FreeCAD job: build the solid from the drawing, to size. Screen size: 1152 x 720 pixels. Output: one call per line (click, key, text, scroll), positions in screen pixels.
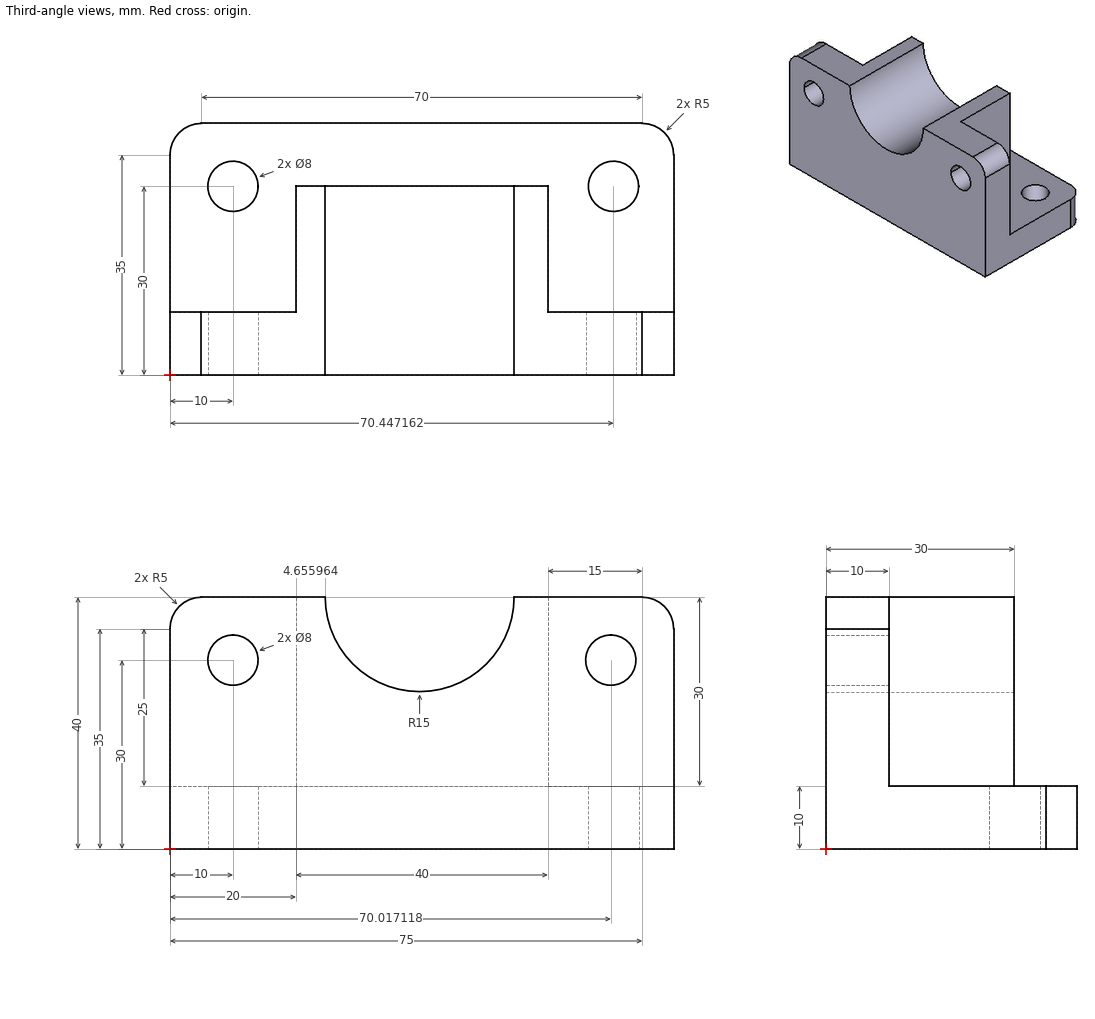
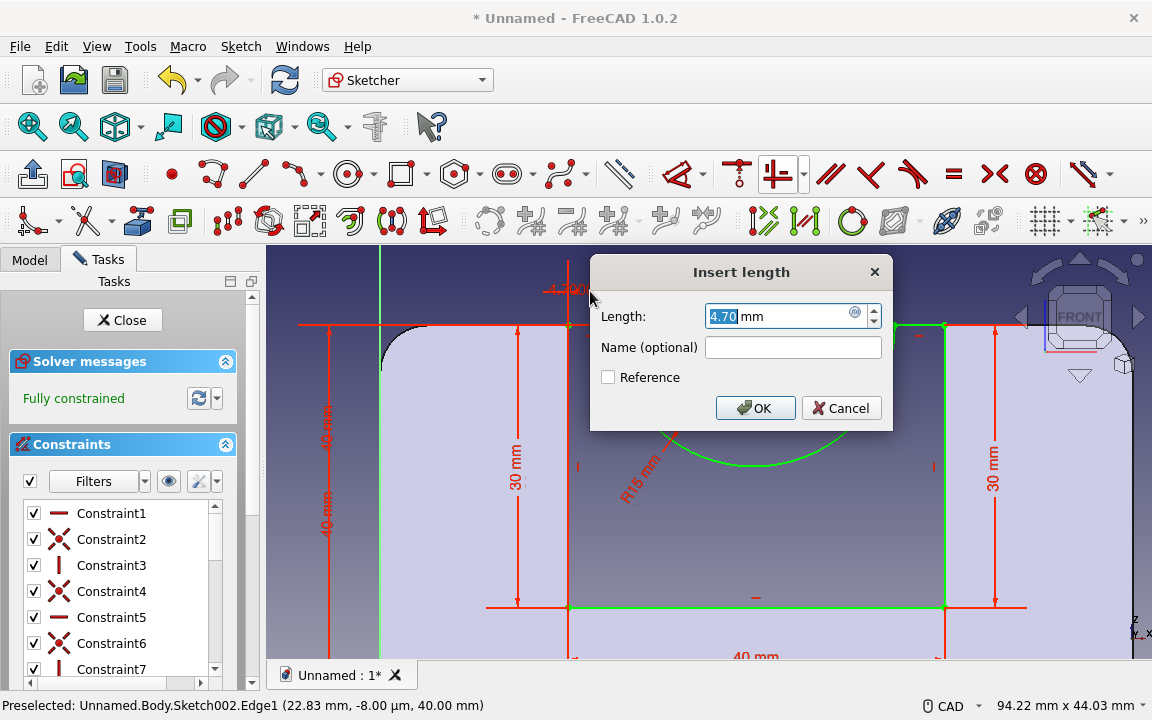
text(4.655964)
key(Return)
key(Escape)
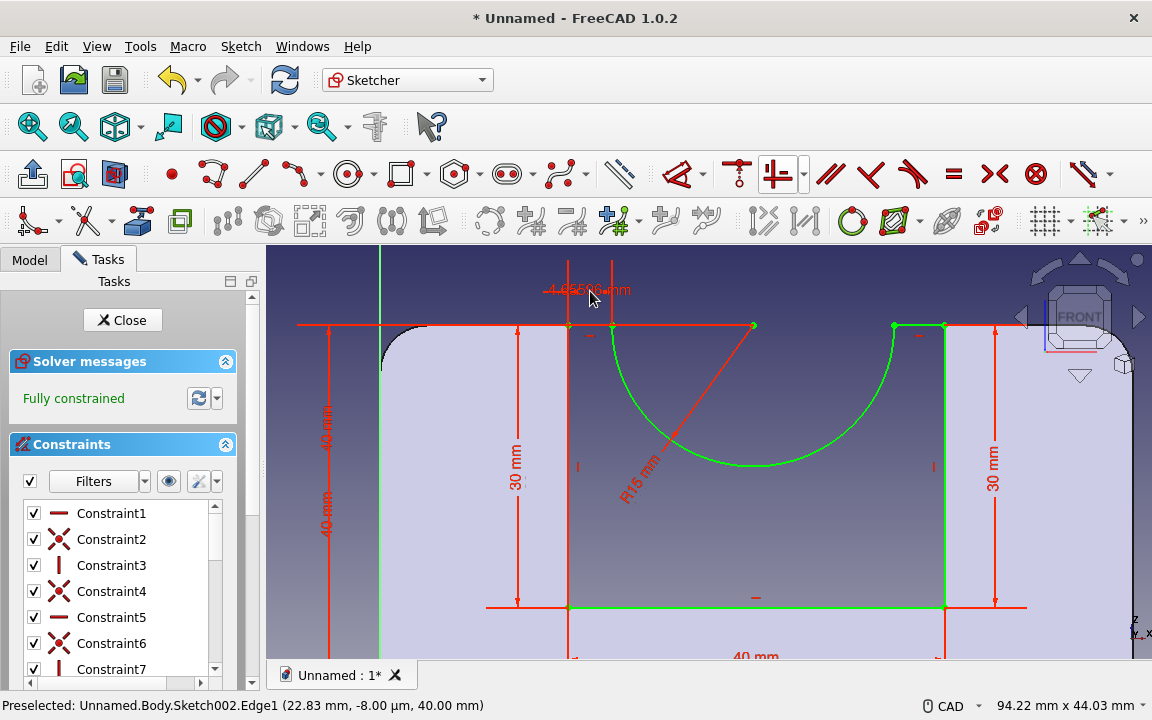
click(123, 320)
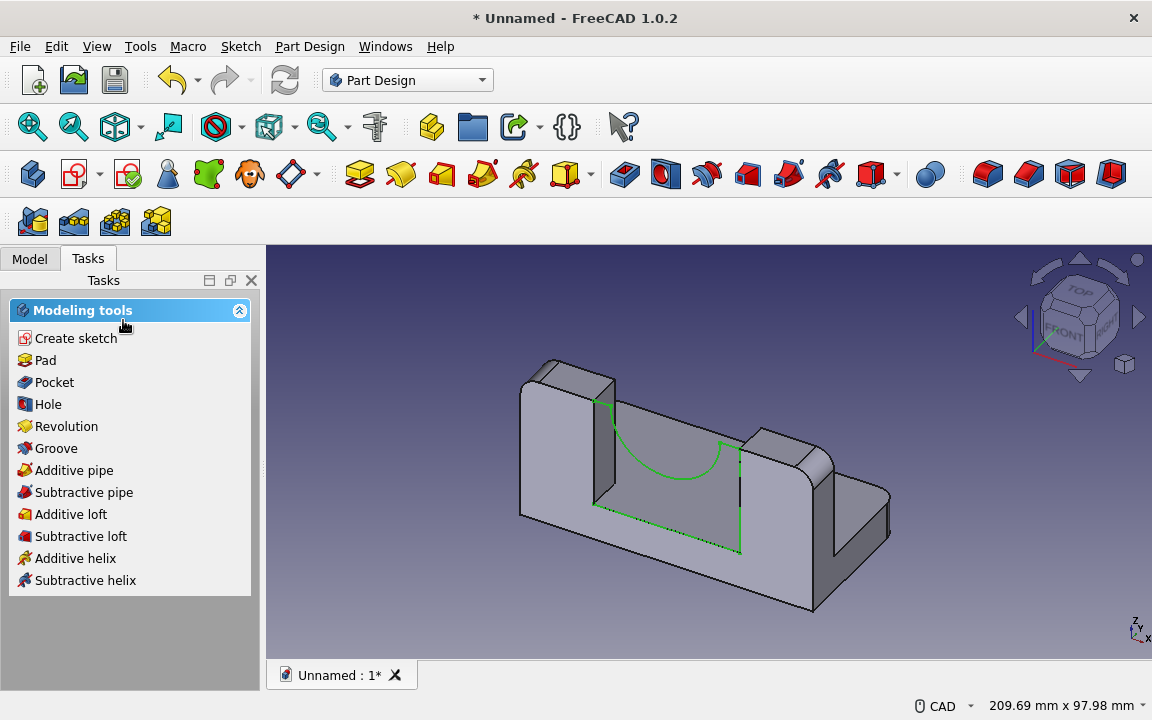
click(360, 174)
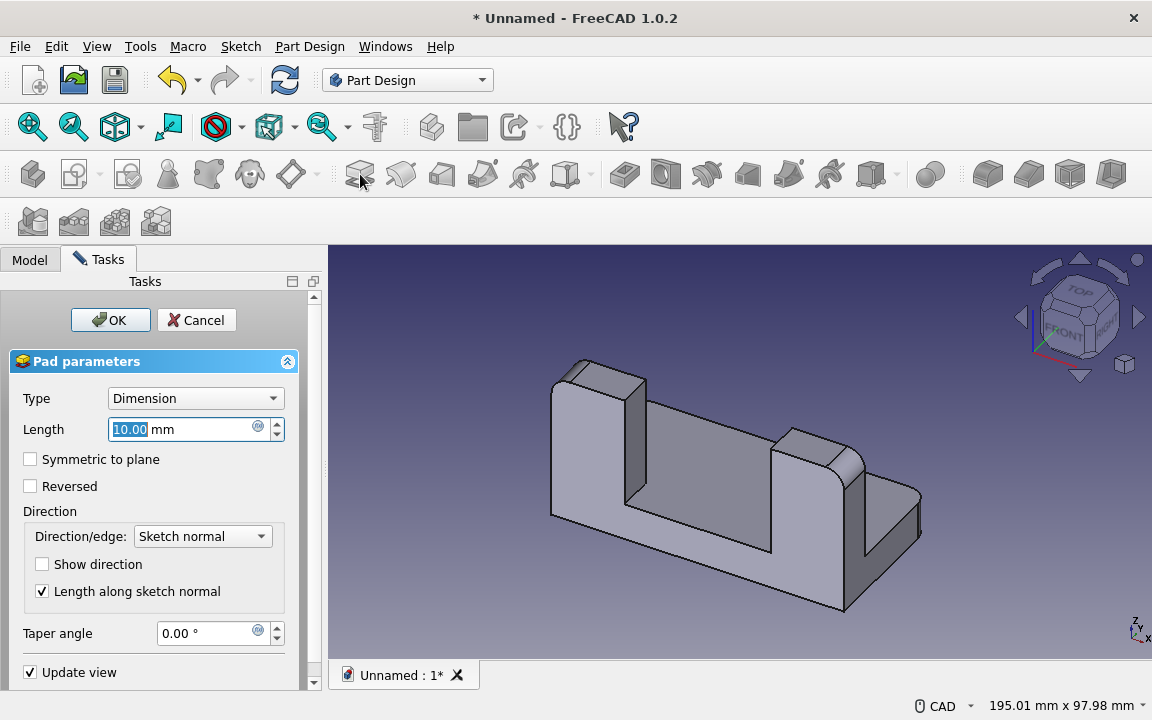
text(30)
key(Tab)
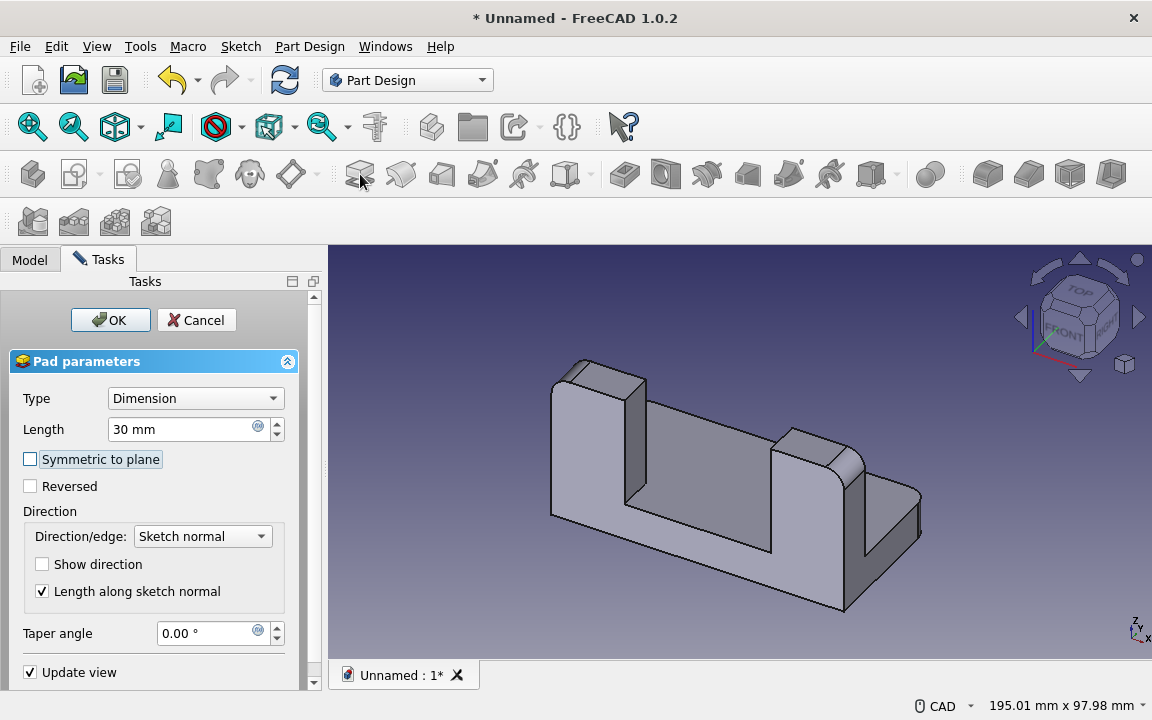
click(31, 486)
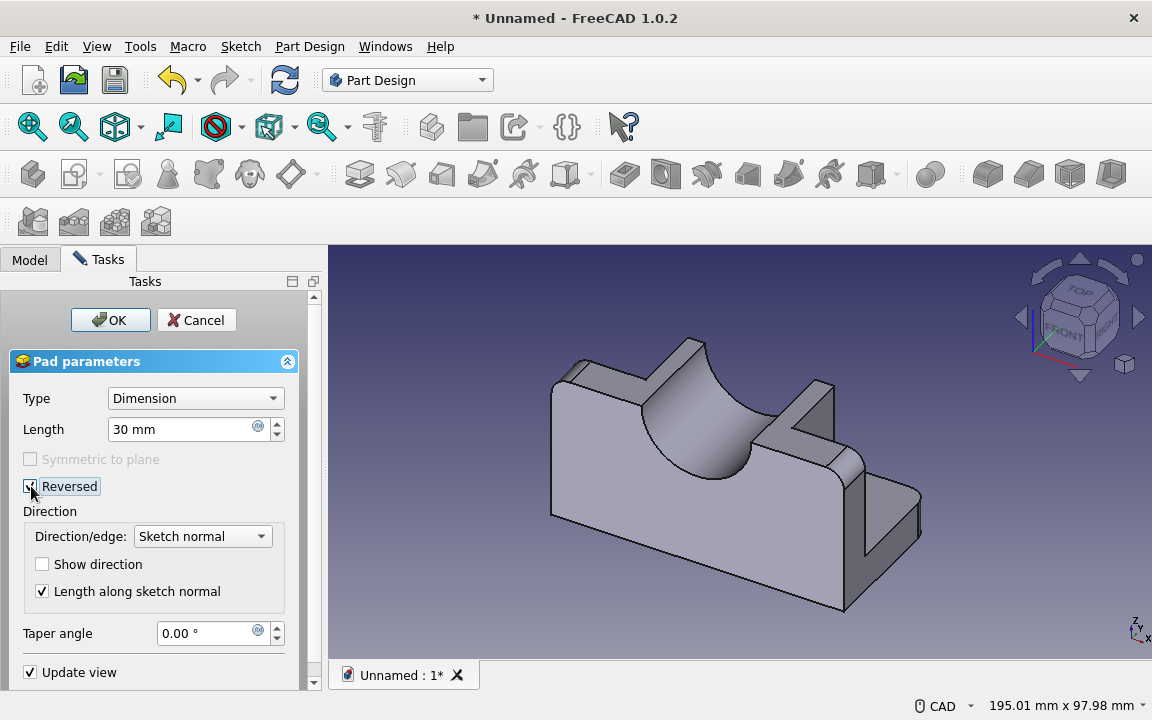
click(111, 320)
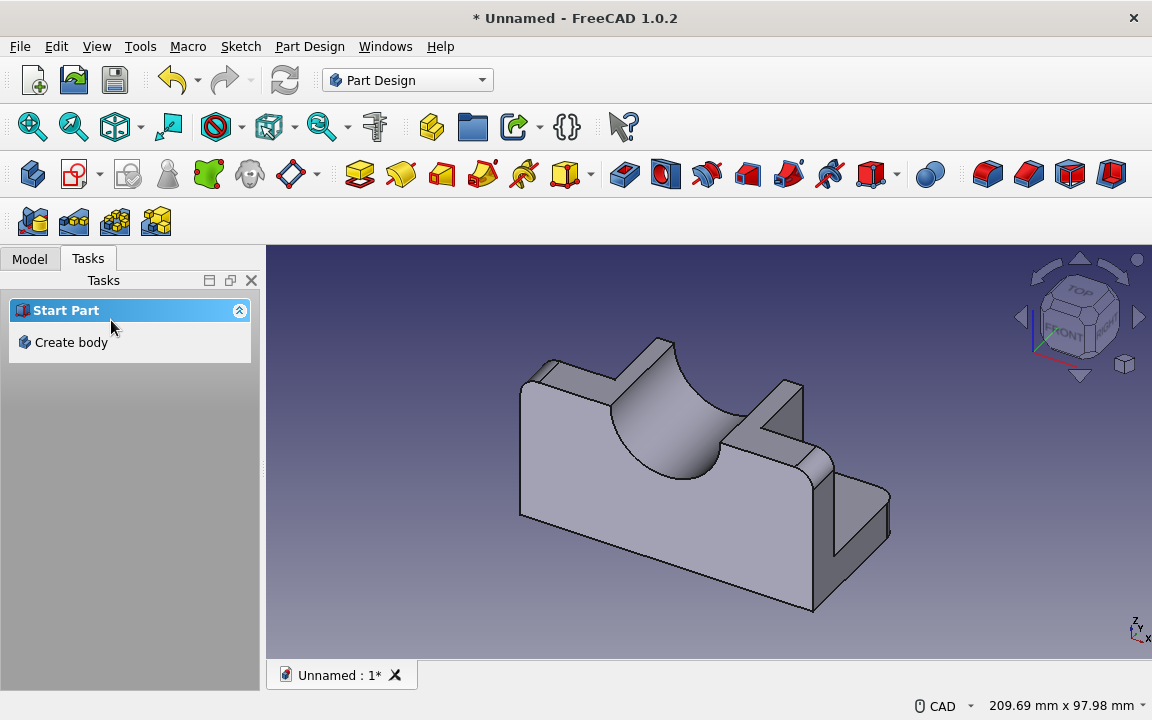
click(863, 499)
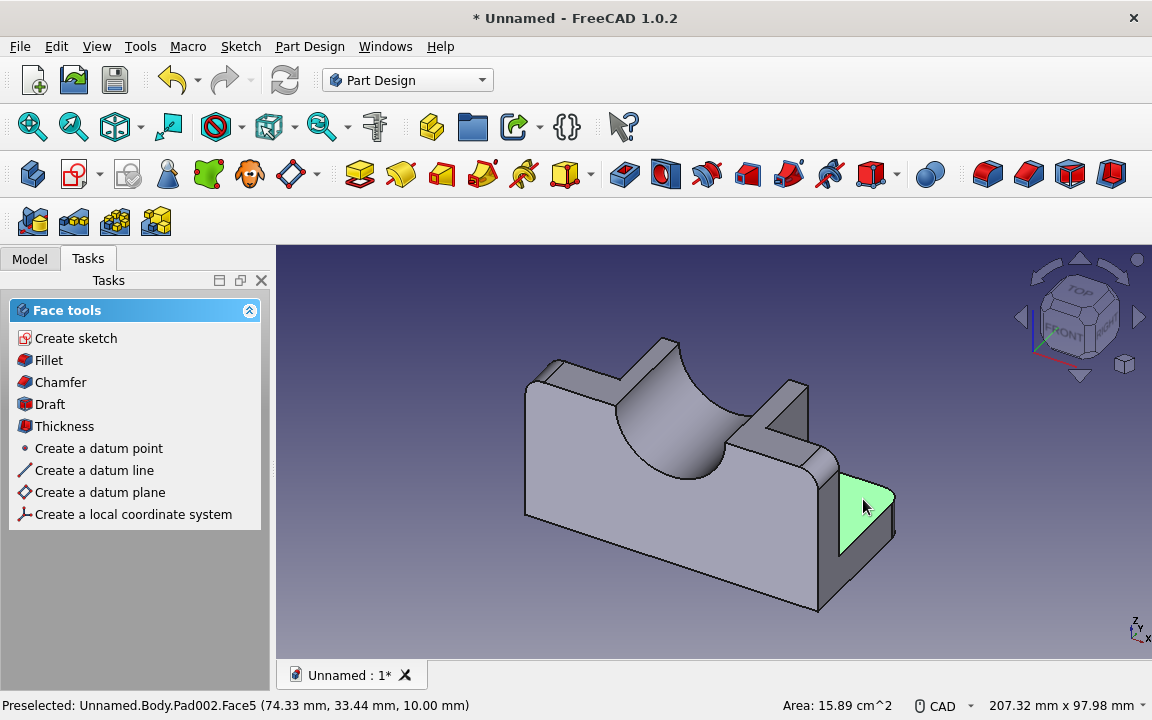
click(74, 174)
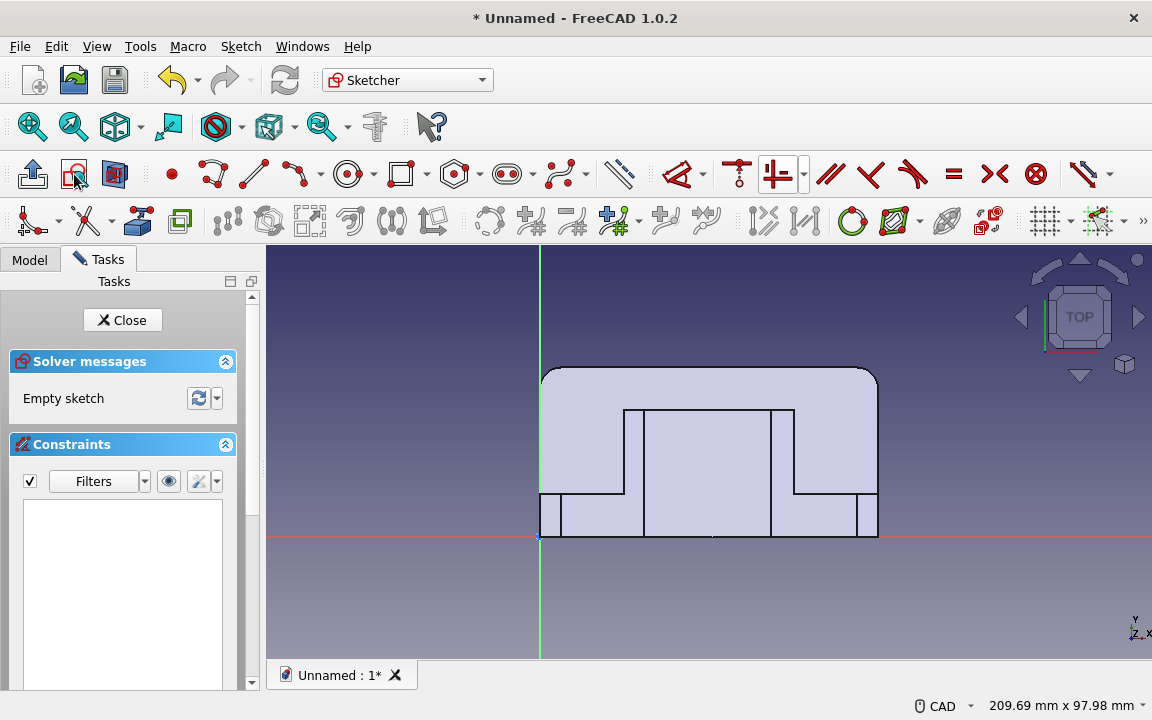
click(115, 174)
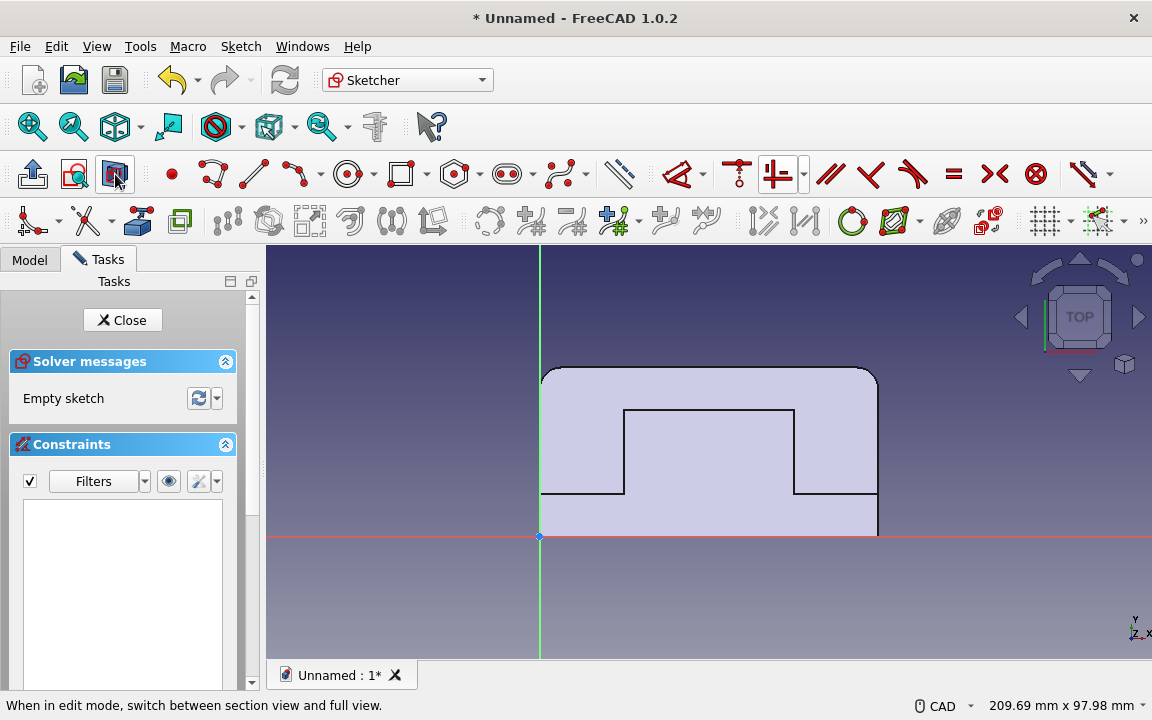
scroll(813, 490, up, 2)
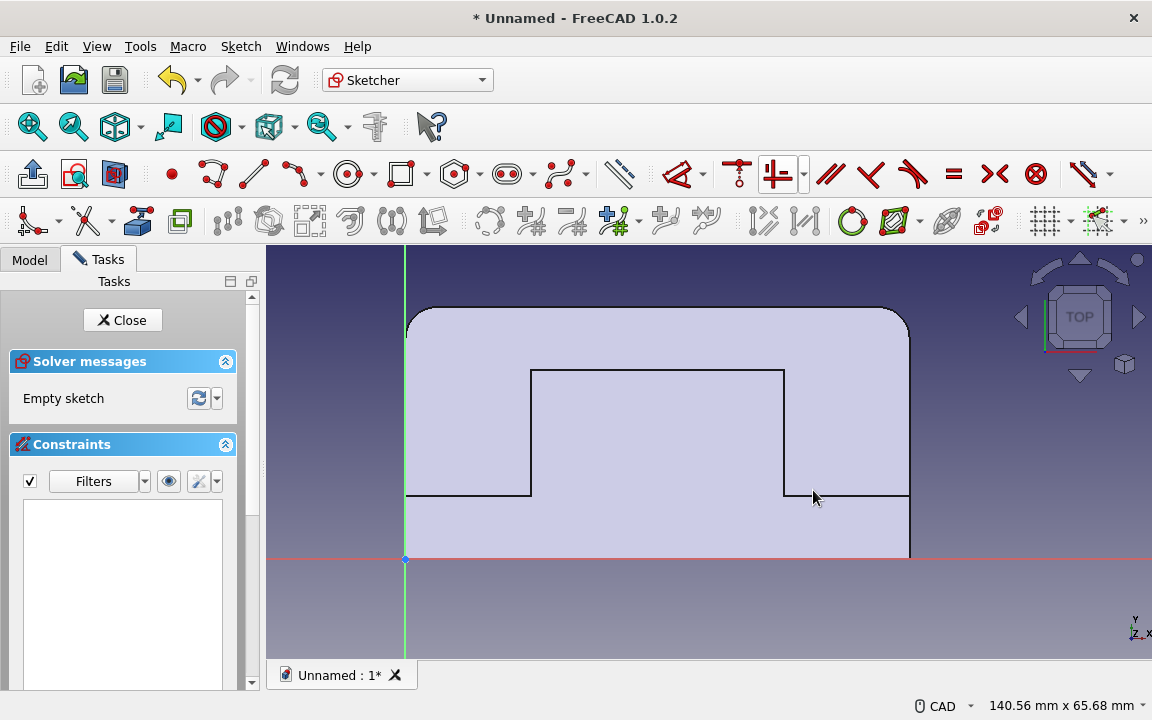
click(348, 174)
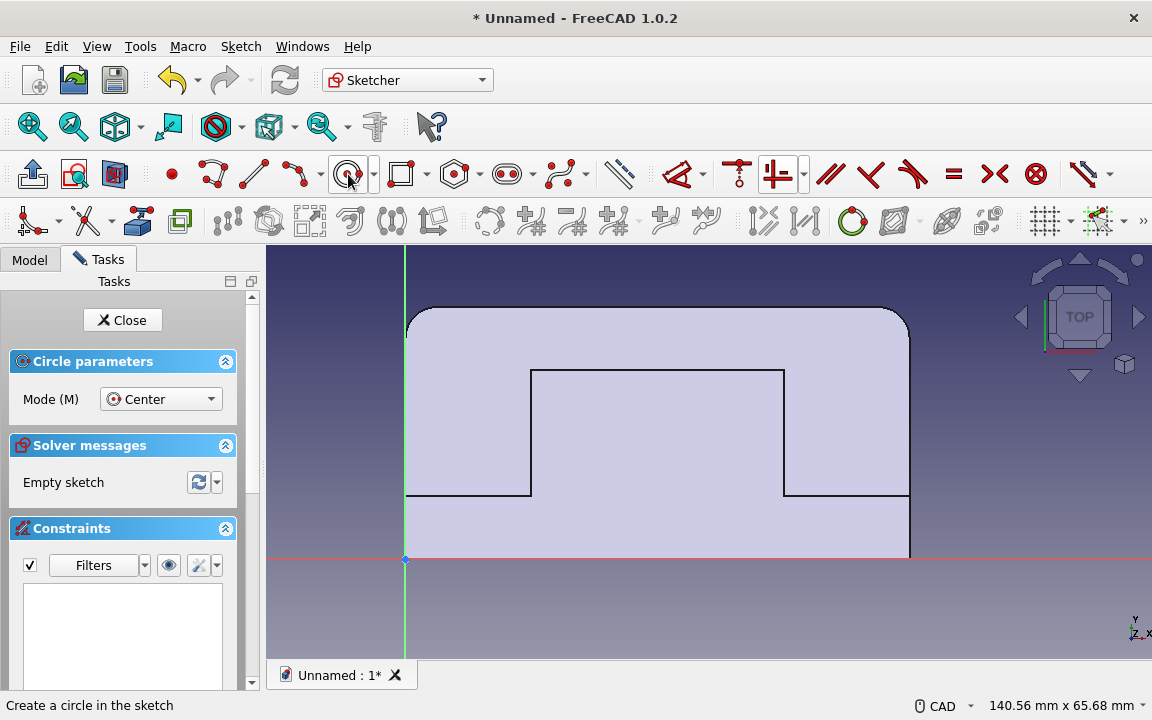
click(468, 370)
click(486, 352)